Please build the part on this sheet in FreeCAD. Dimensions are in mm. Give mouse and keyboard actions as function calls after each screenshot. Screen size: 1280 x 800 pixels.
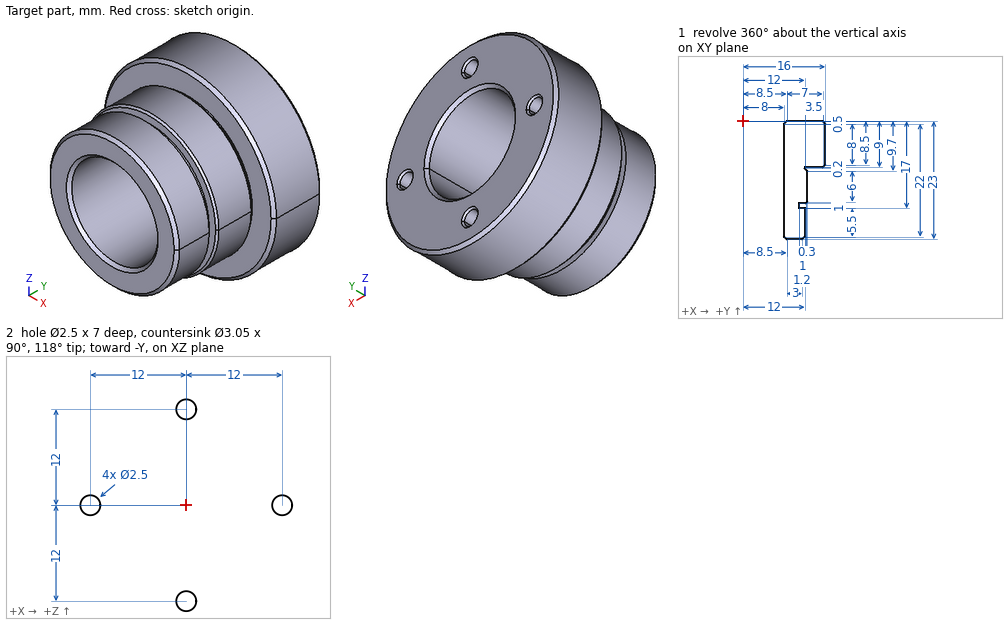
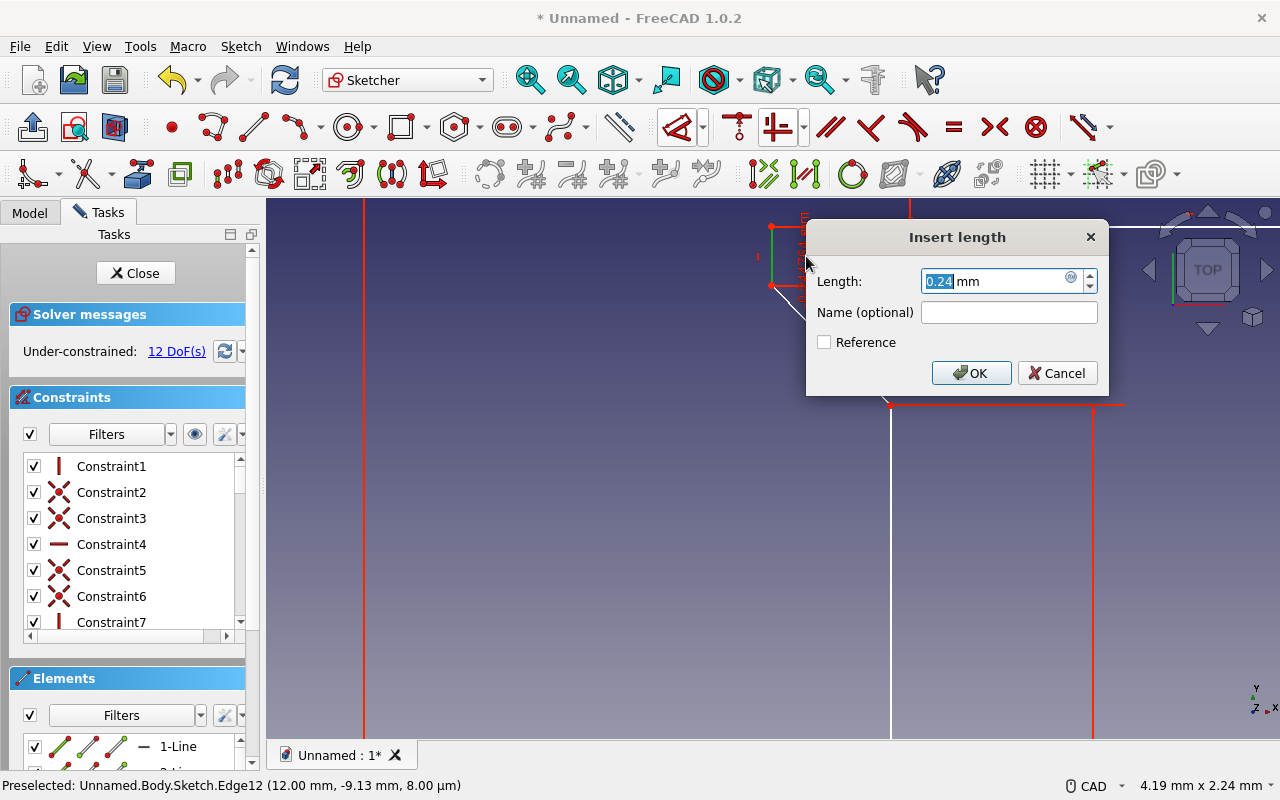
text(0.2)
key(Return)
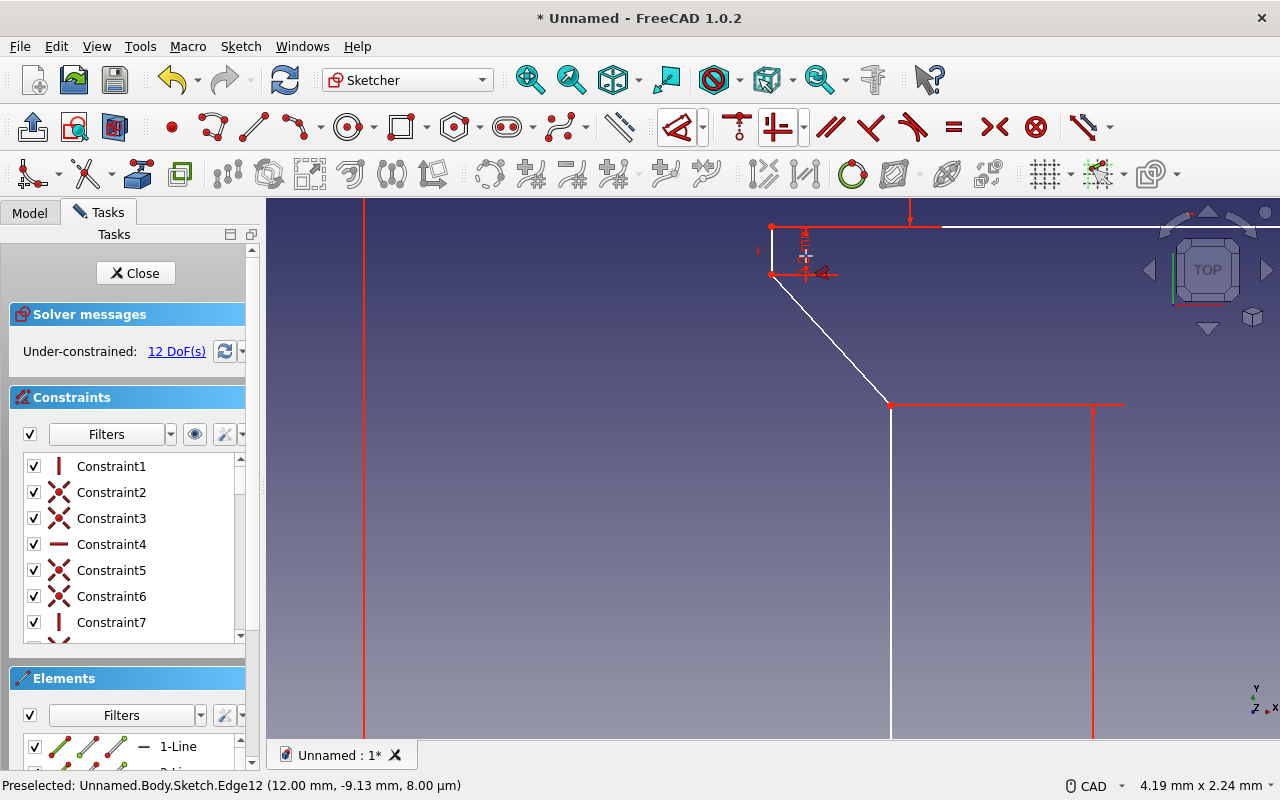
scroll(763, 445, down, 14)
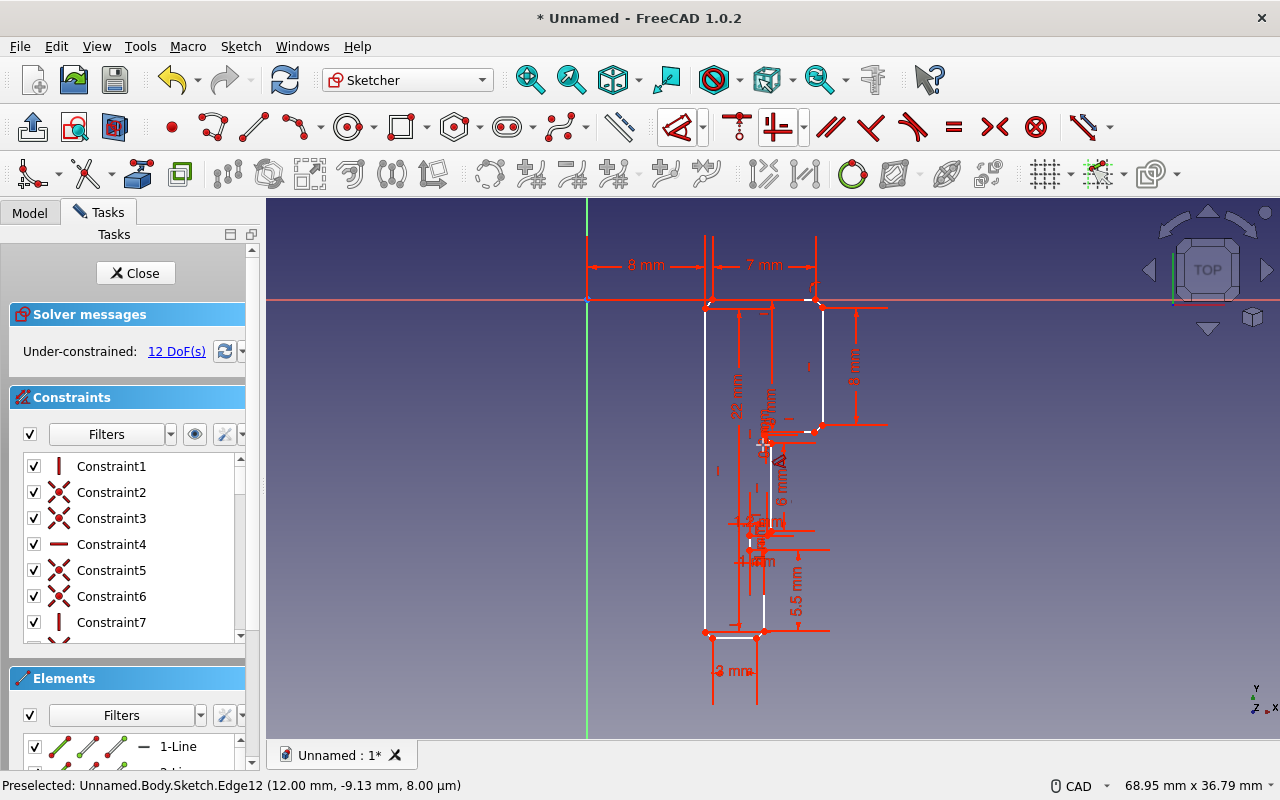
click(779, 432)
click(789, 466)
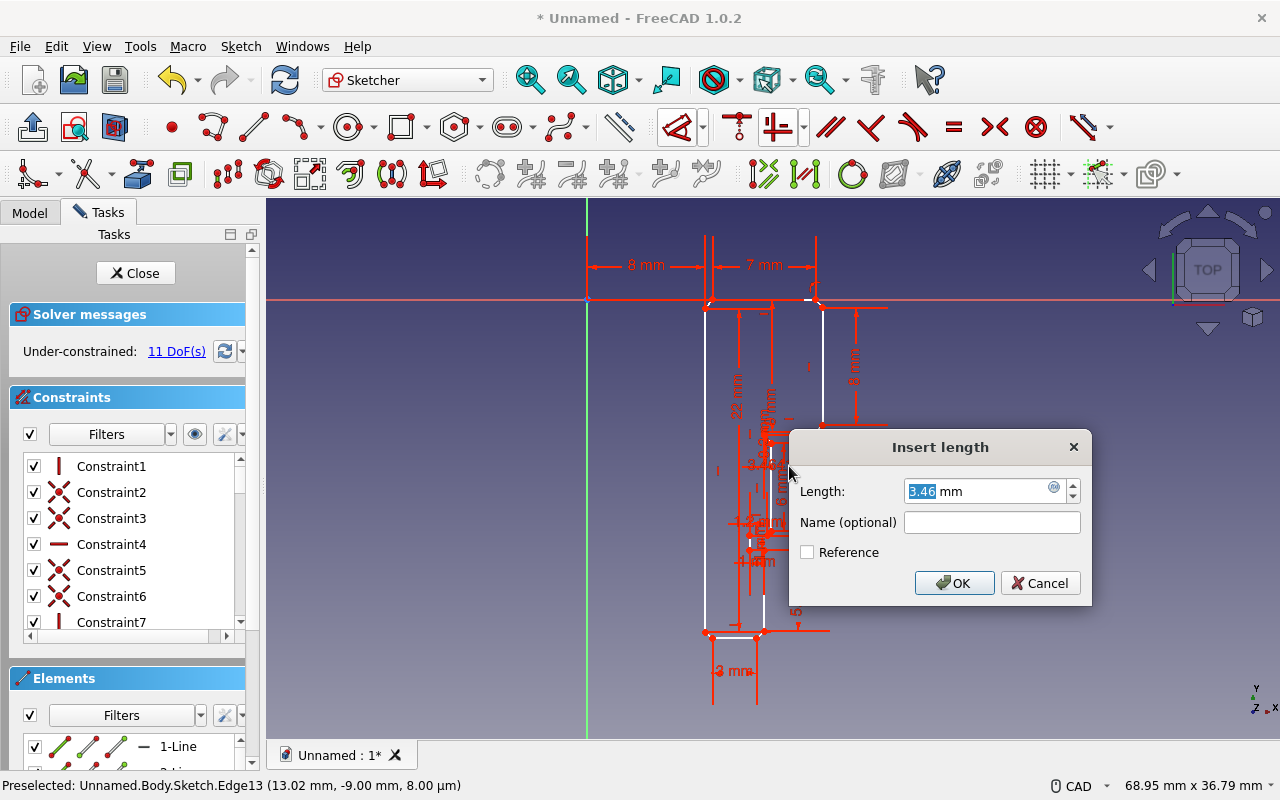
text(3.5)
key(Return)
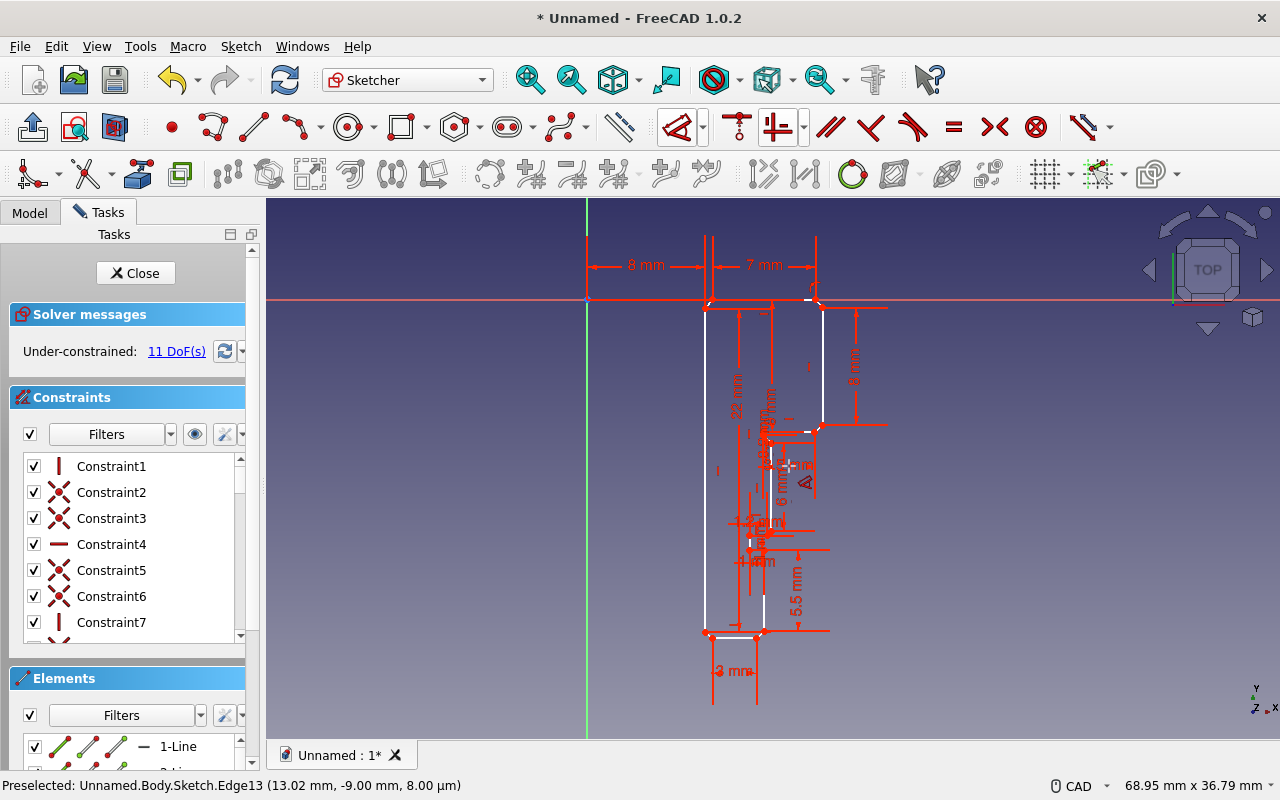
scroll(713, 638, up, 2)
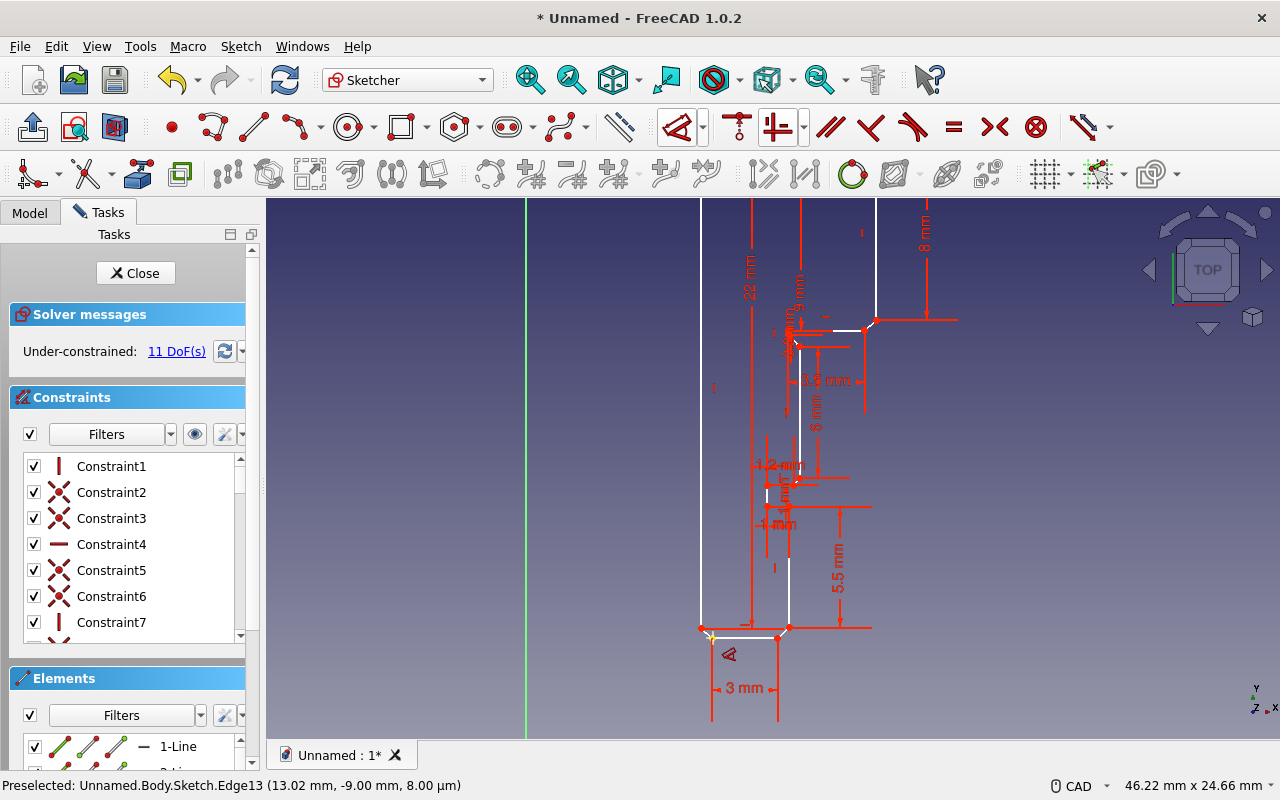
click(712, 638)
click(492, 432)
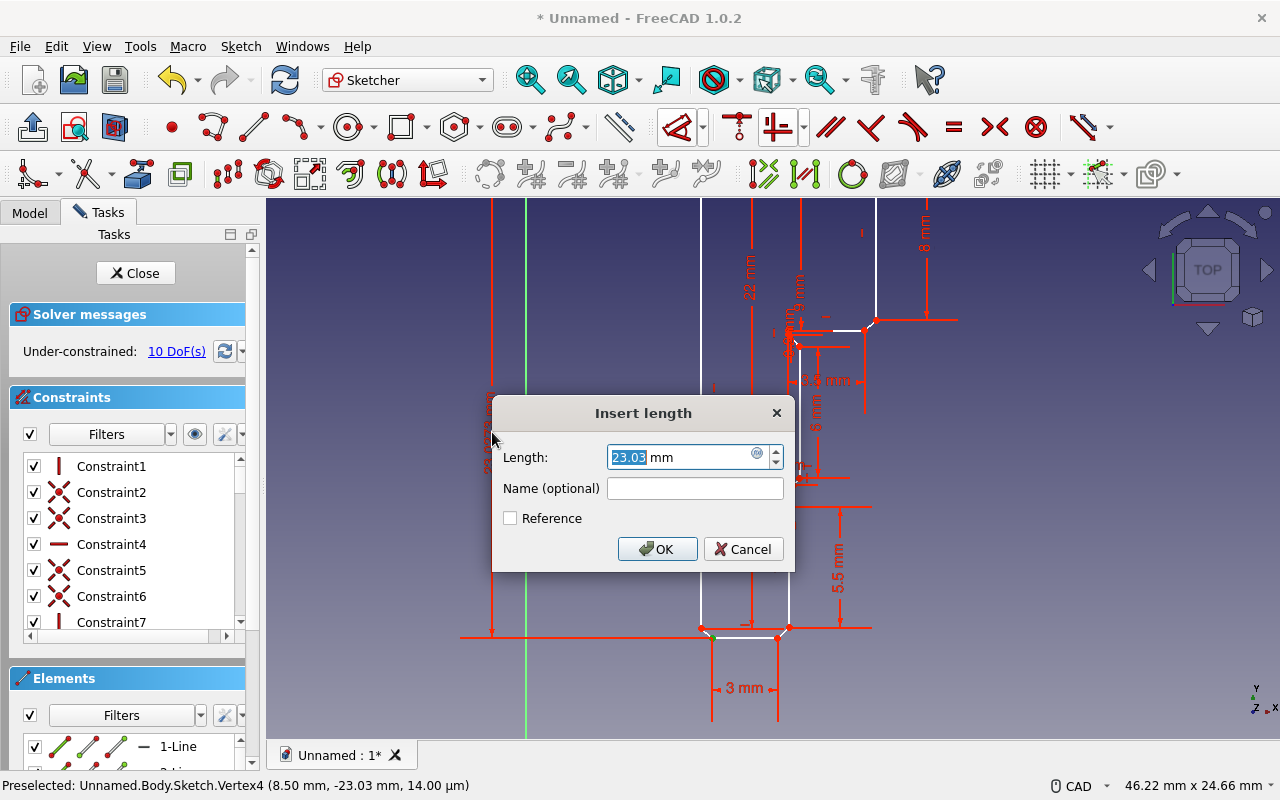
text(23)
key(Return)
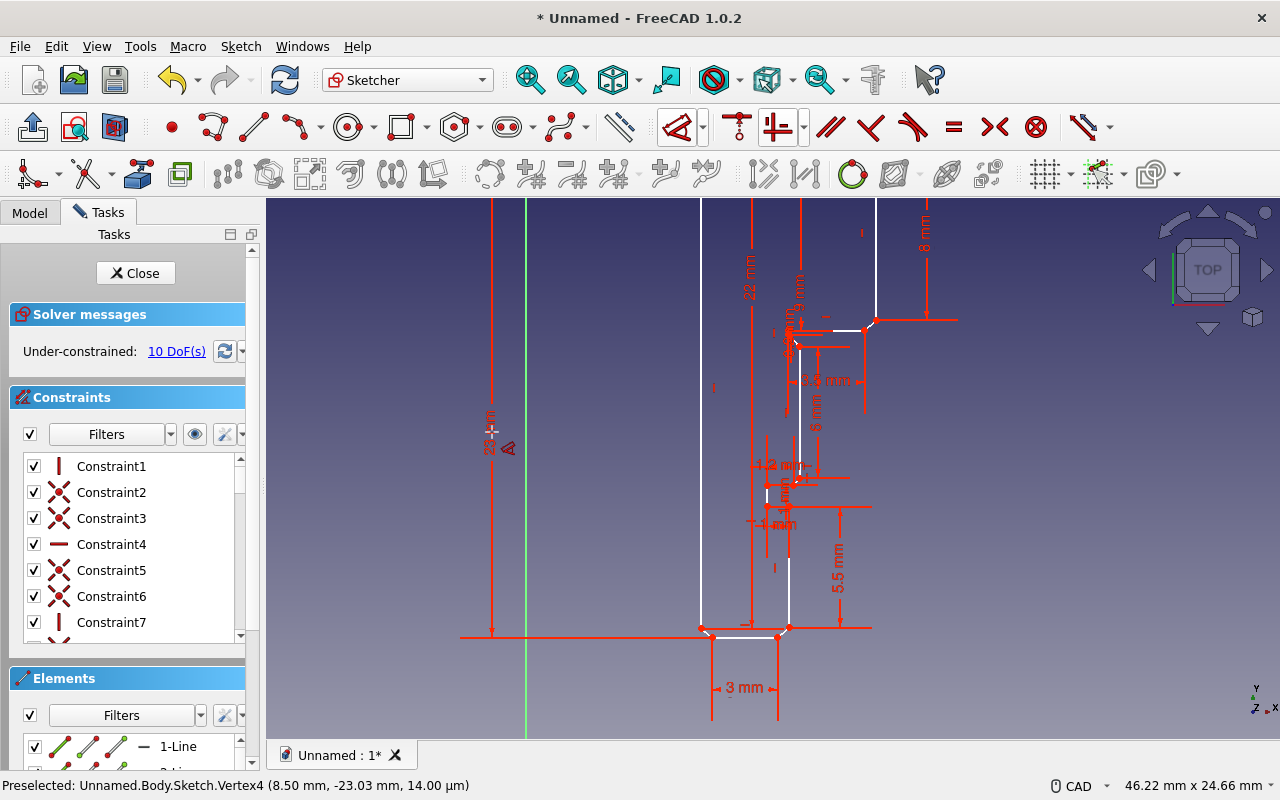
click(789, 628)
click(657, 662)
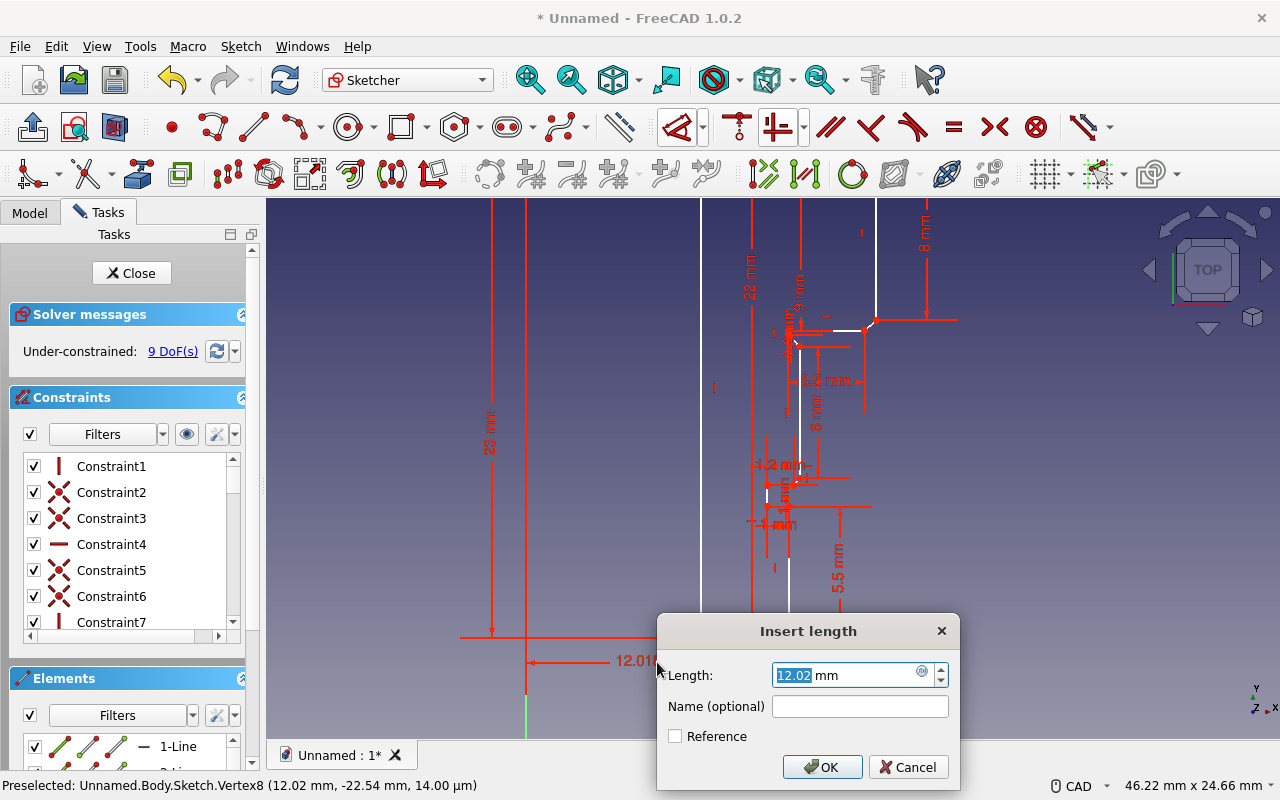
text(12)
key(Return)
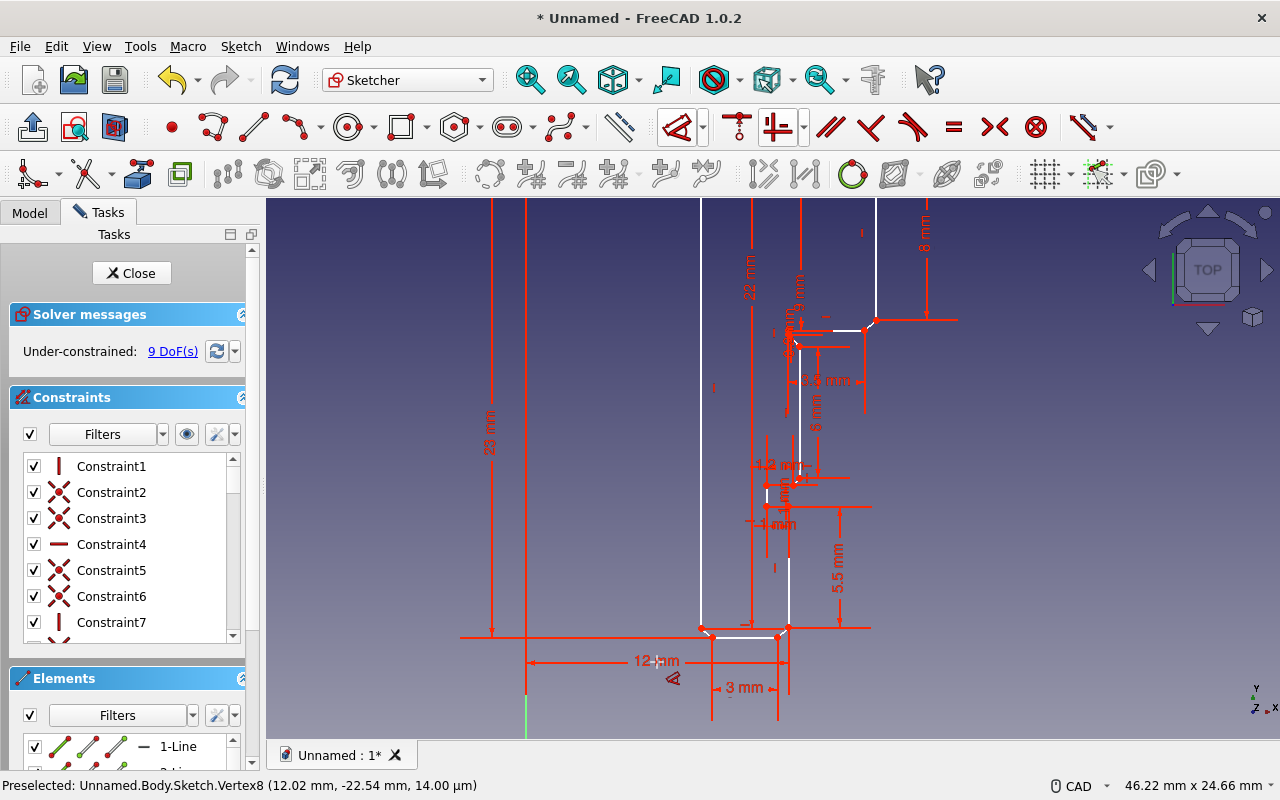
click(789, 507)
click(492, 366)